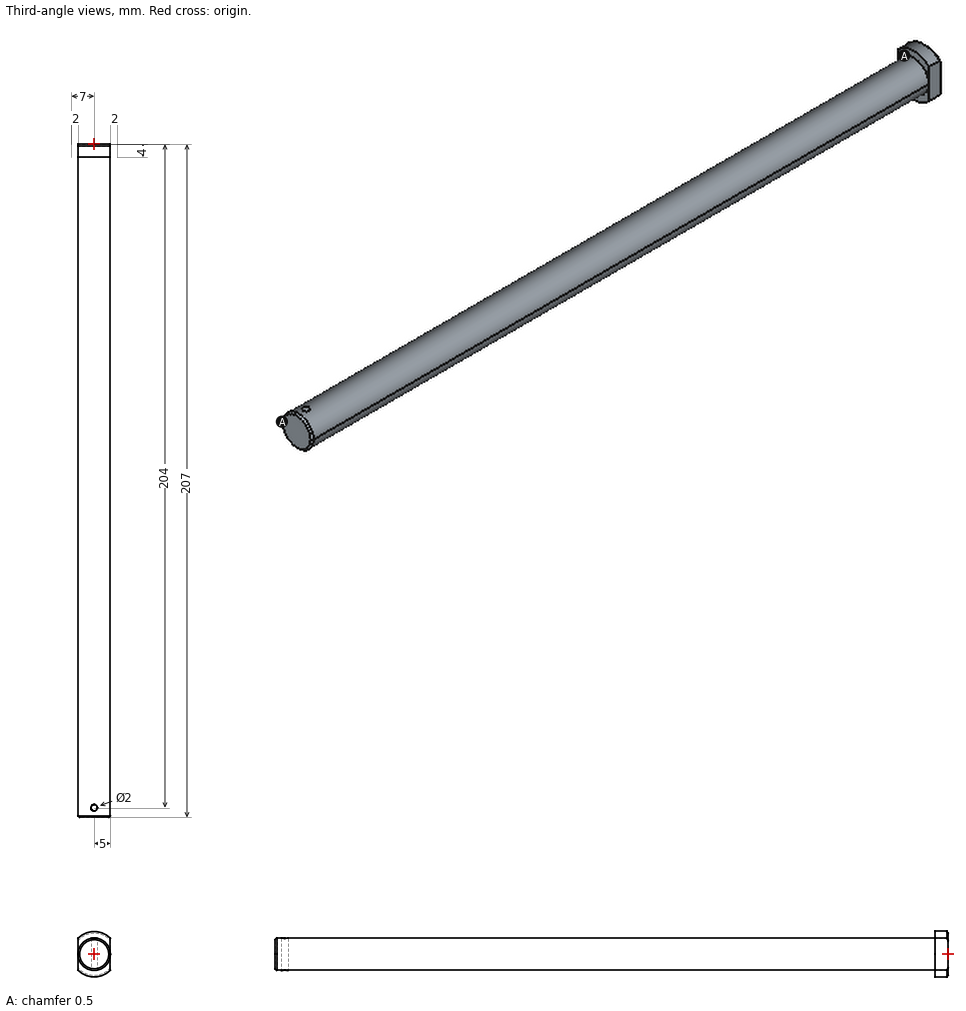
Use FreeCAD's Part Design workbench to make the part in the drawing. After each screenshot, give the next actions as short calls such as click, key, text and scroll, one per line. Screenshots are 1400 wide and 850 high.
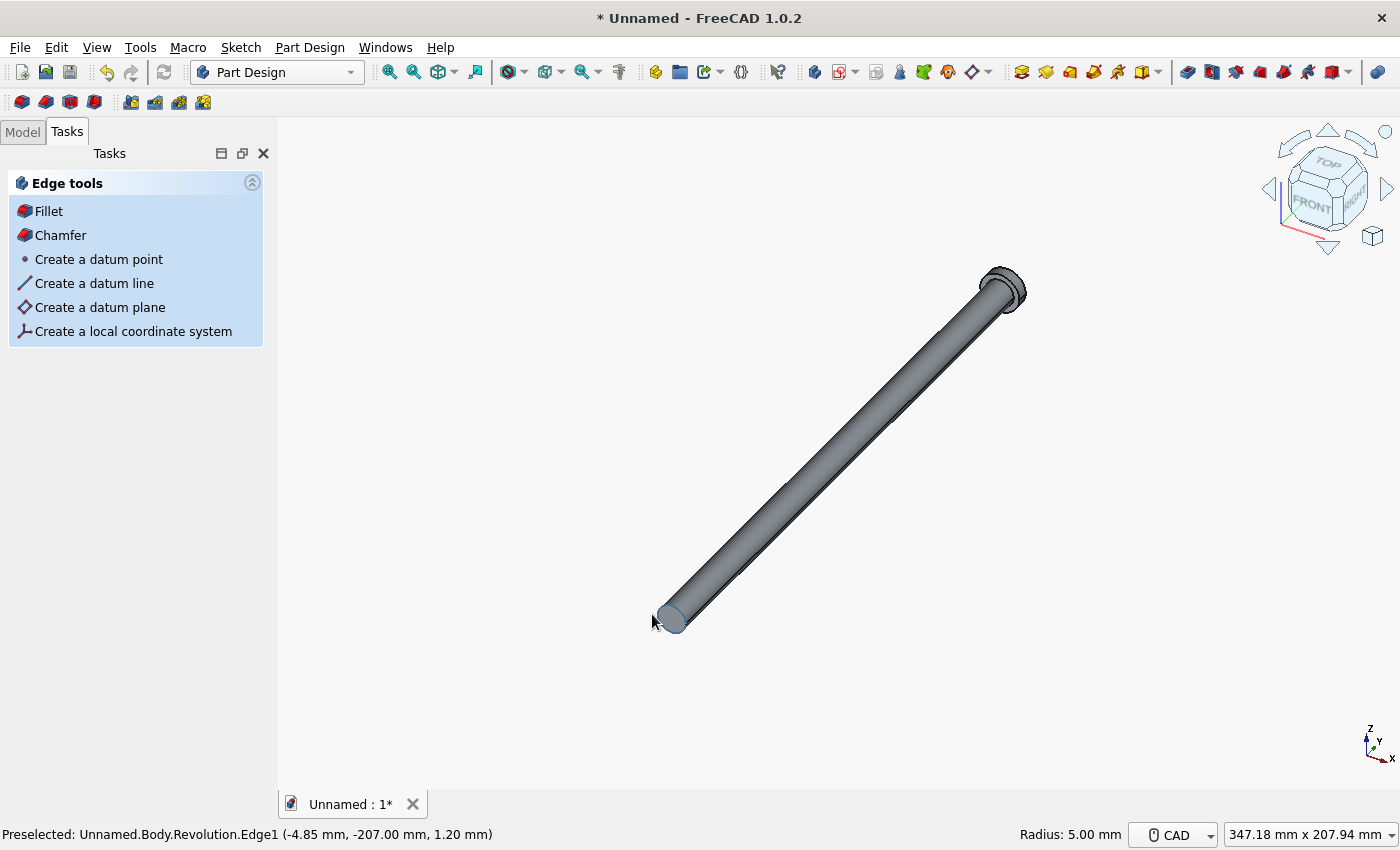
key(0)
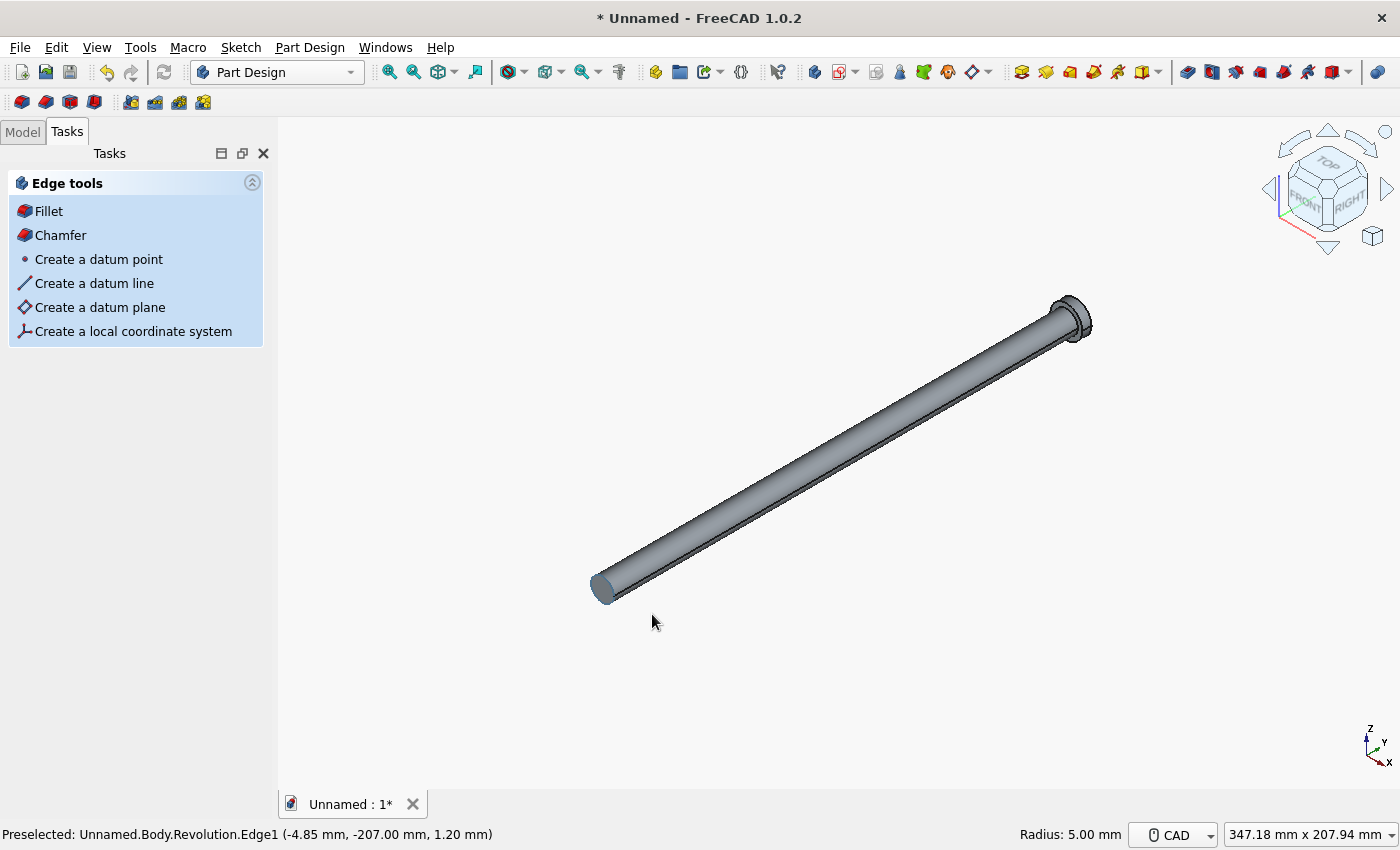
click(1071, 295, ctrl)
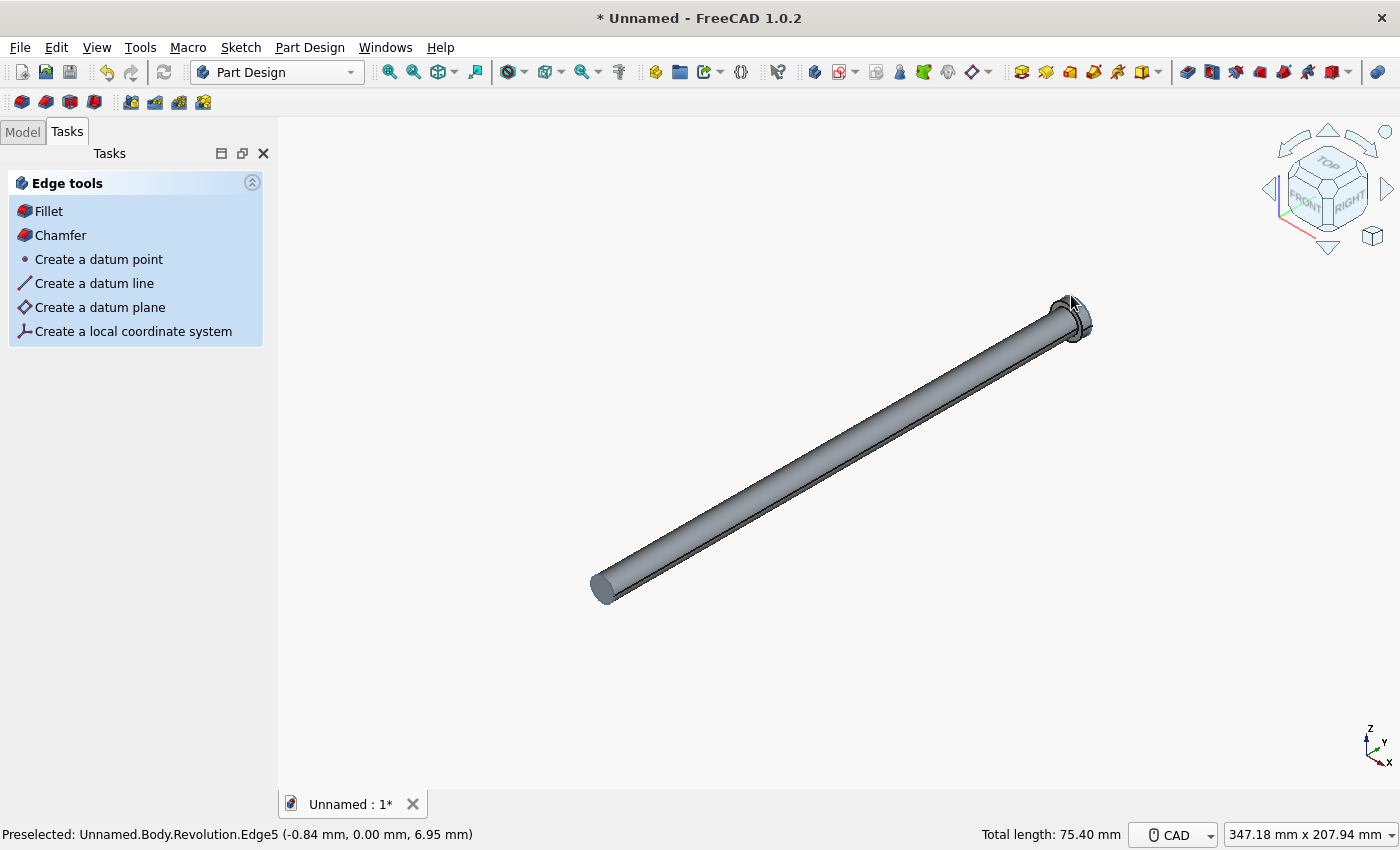
click(46, 102)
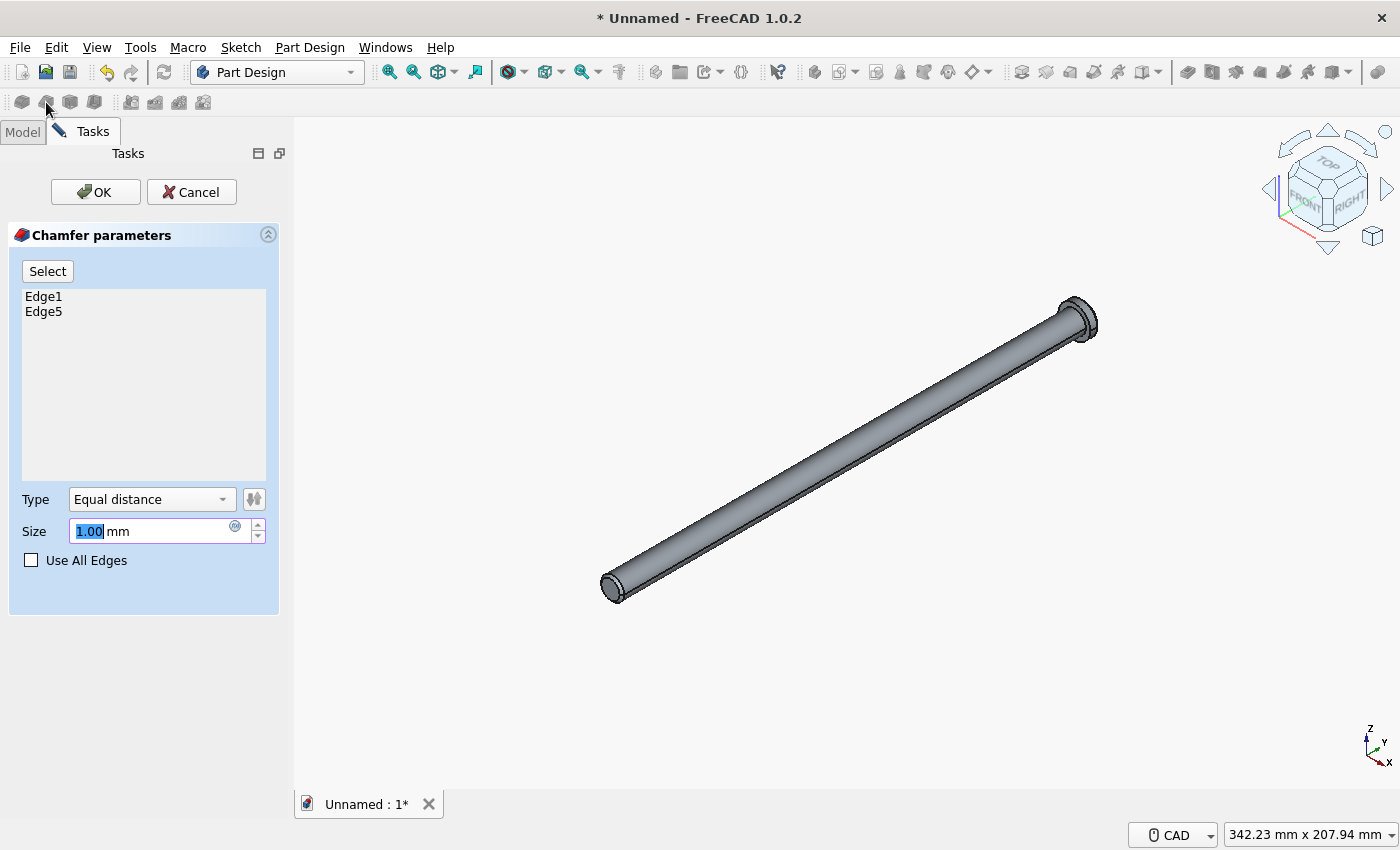
text(0.5)
key(Tab)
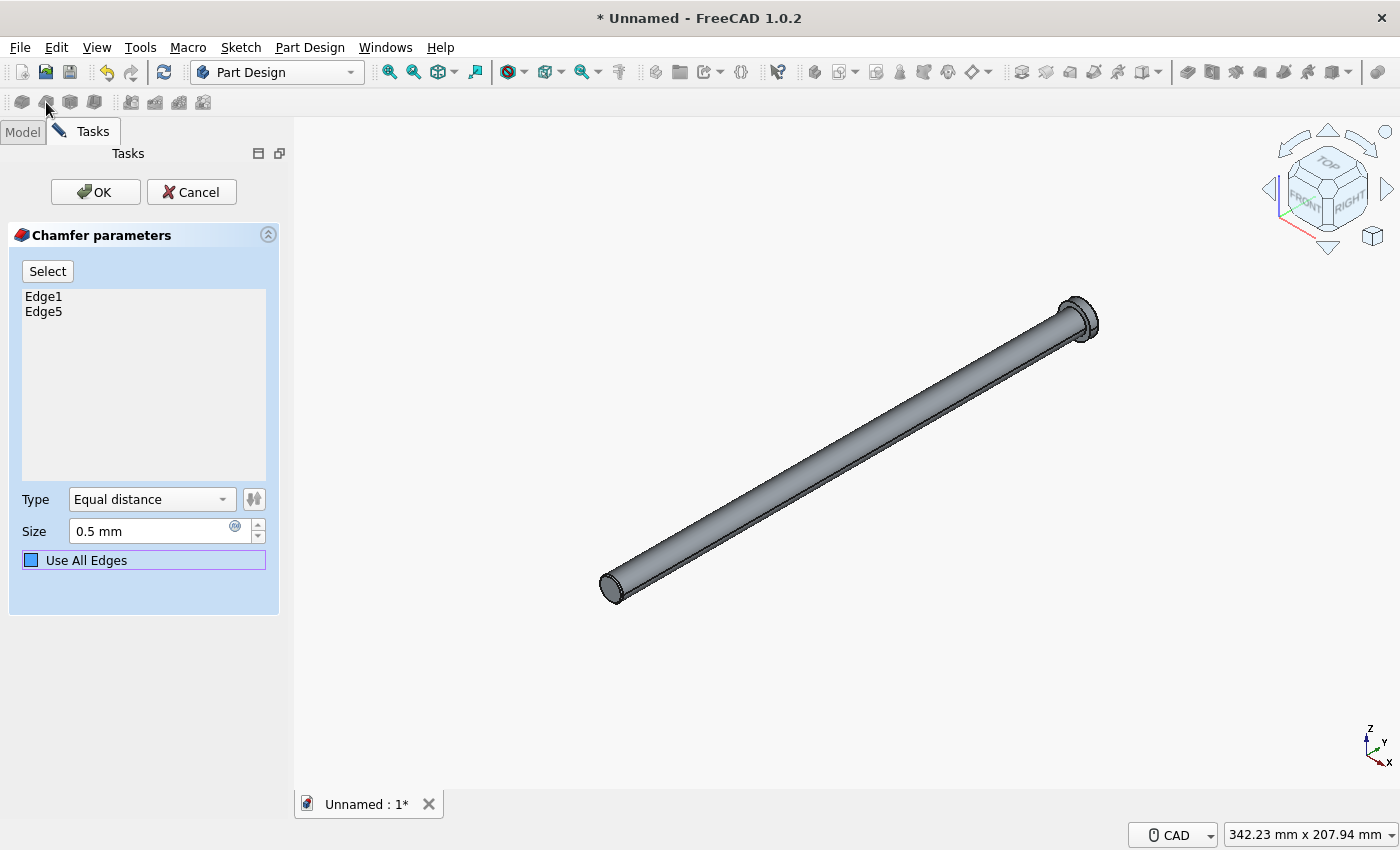
click(96, 192)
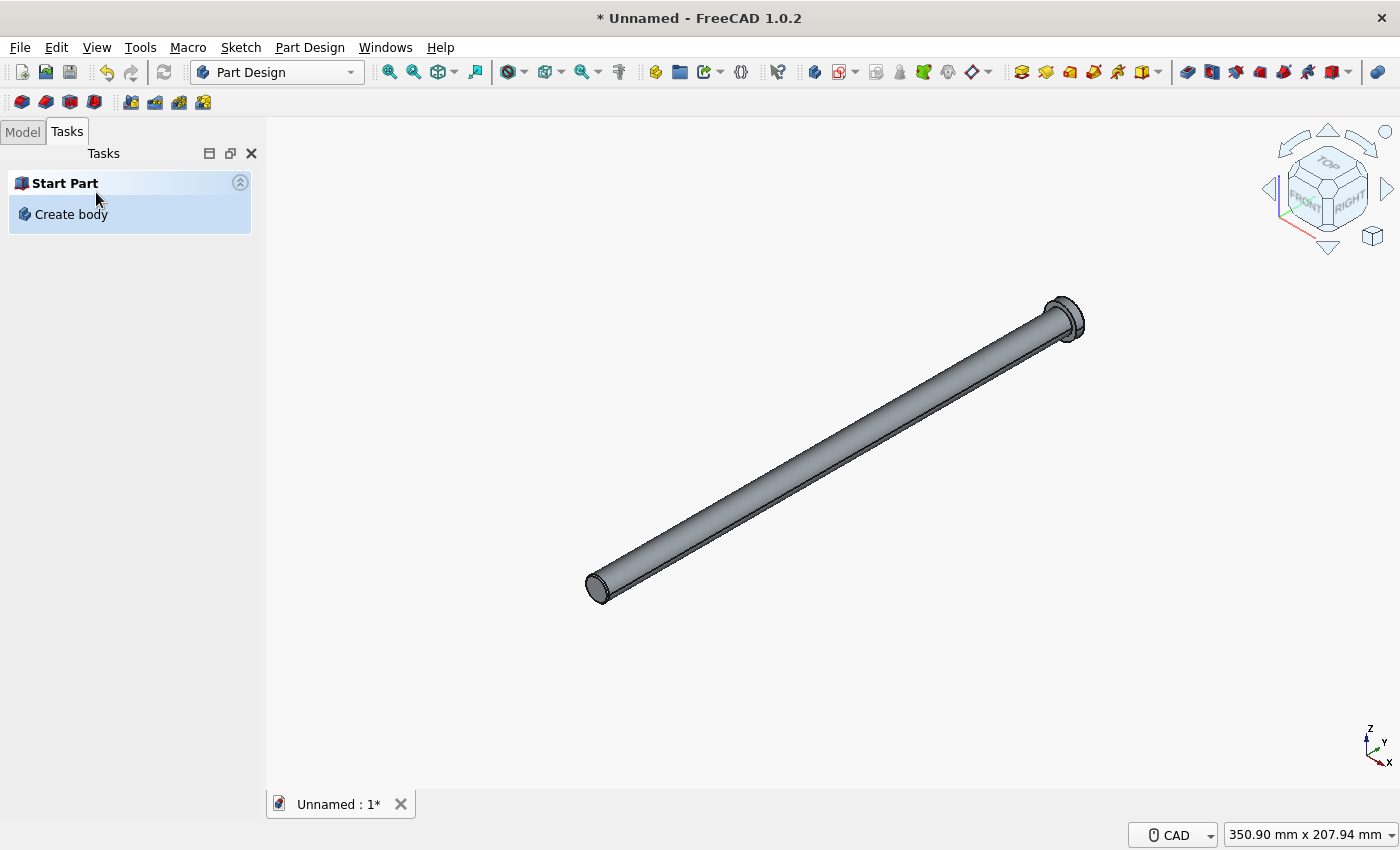
click(840, 72)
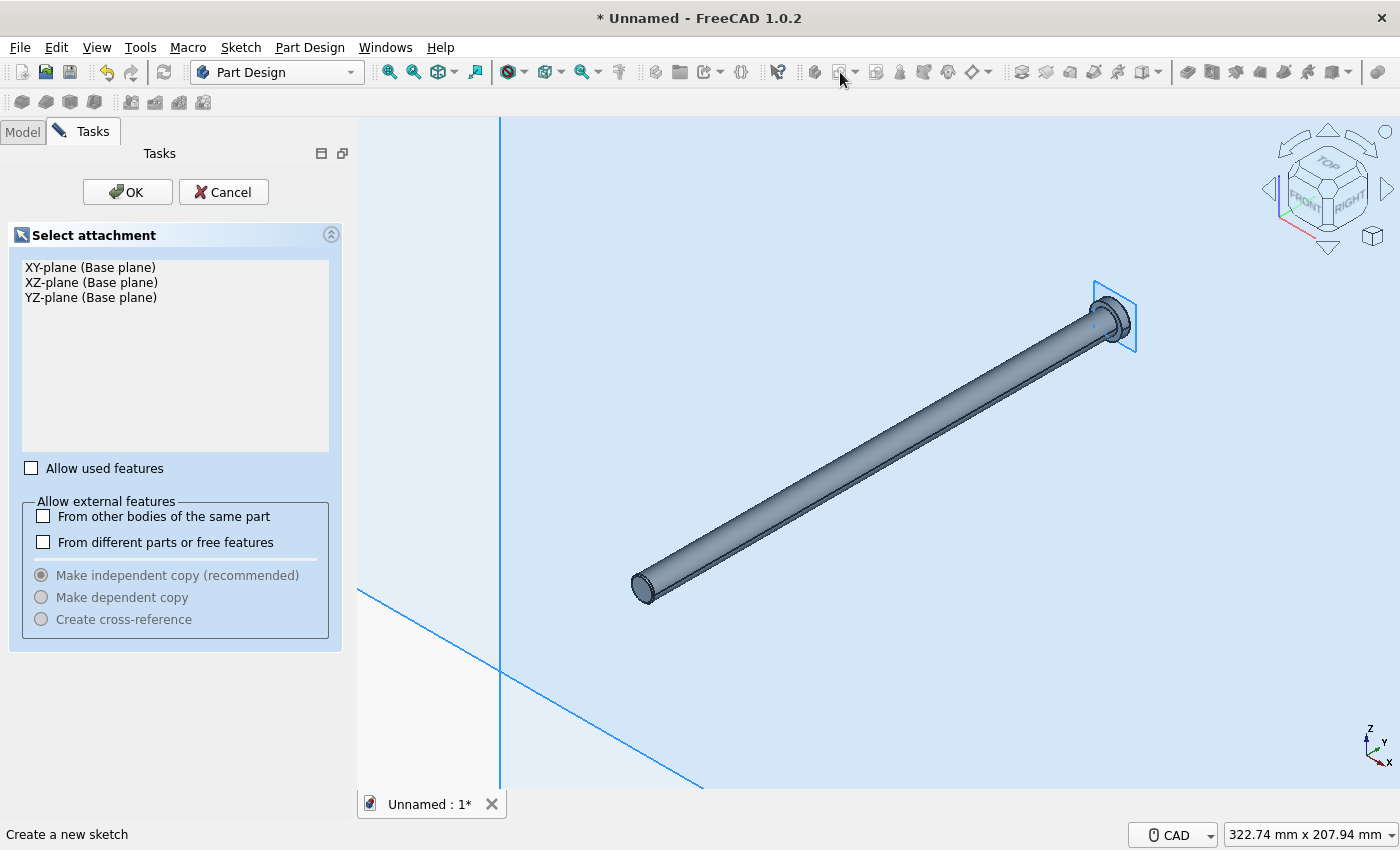
click(82, 268)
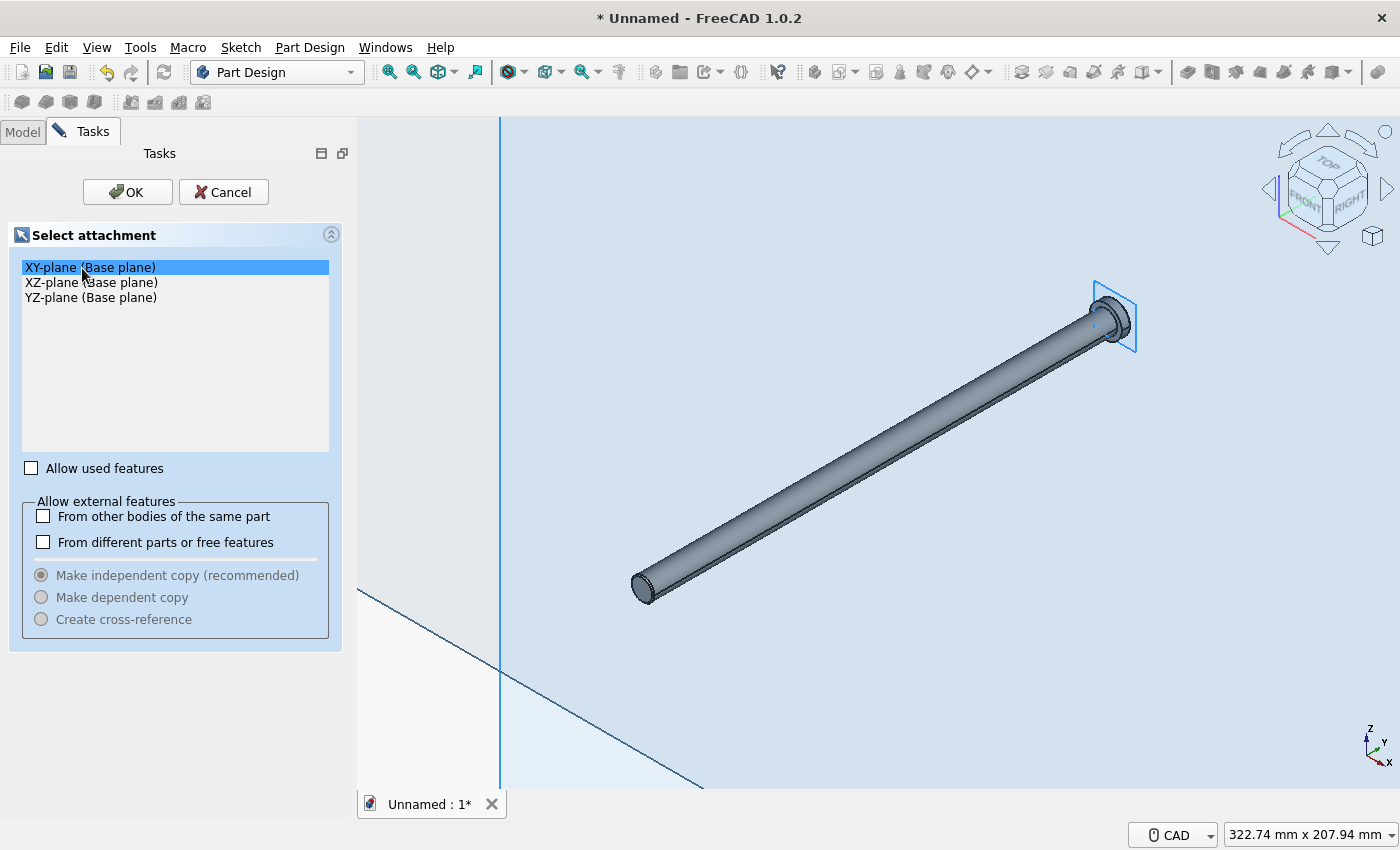
click(128, 192)